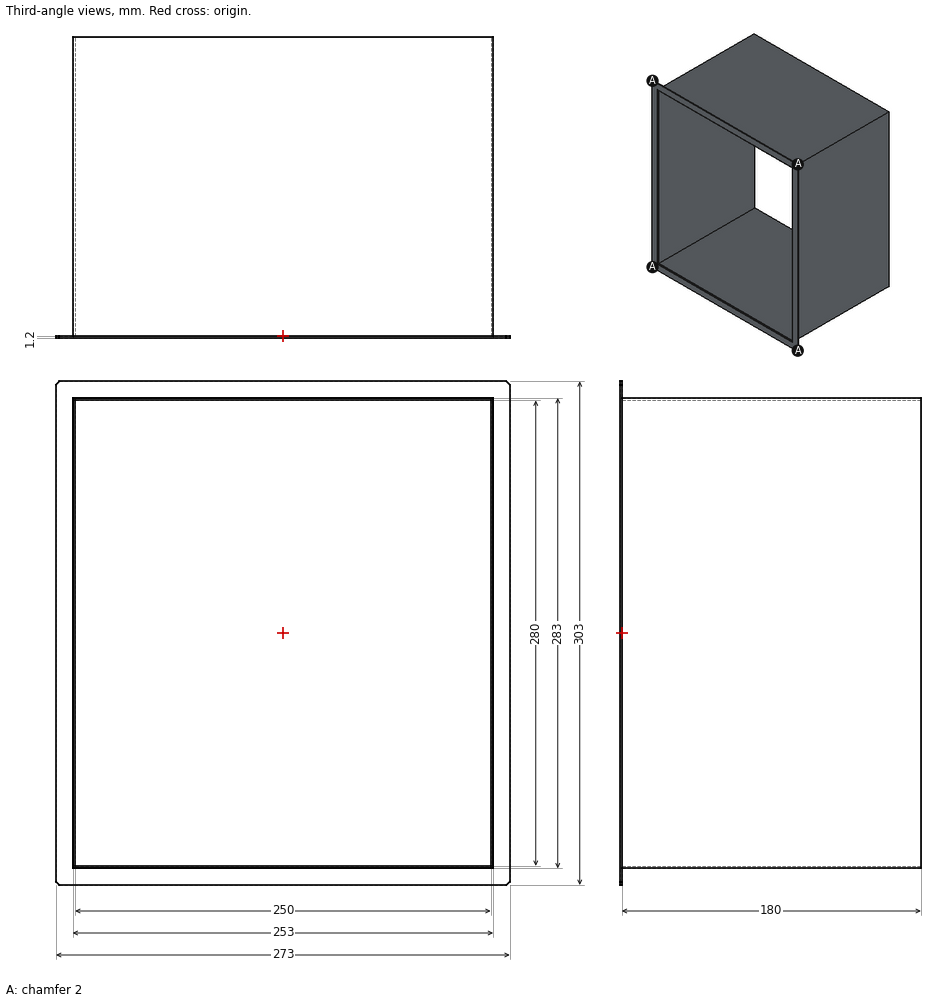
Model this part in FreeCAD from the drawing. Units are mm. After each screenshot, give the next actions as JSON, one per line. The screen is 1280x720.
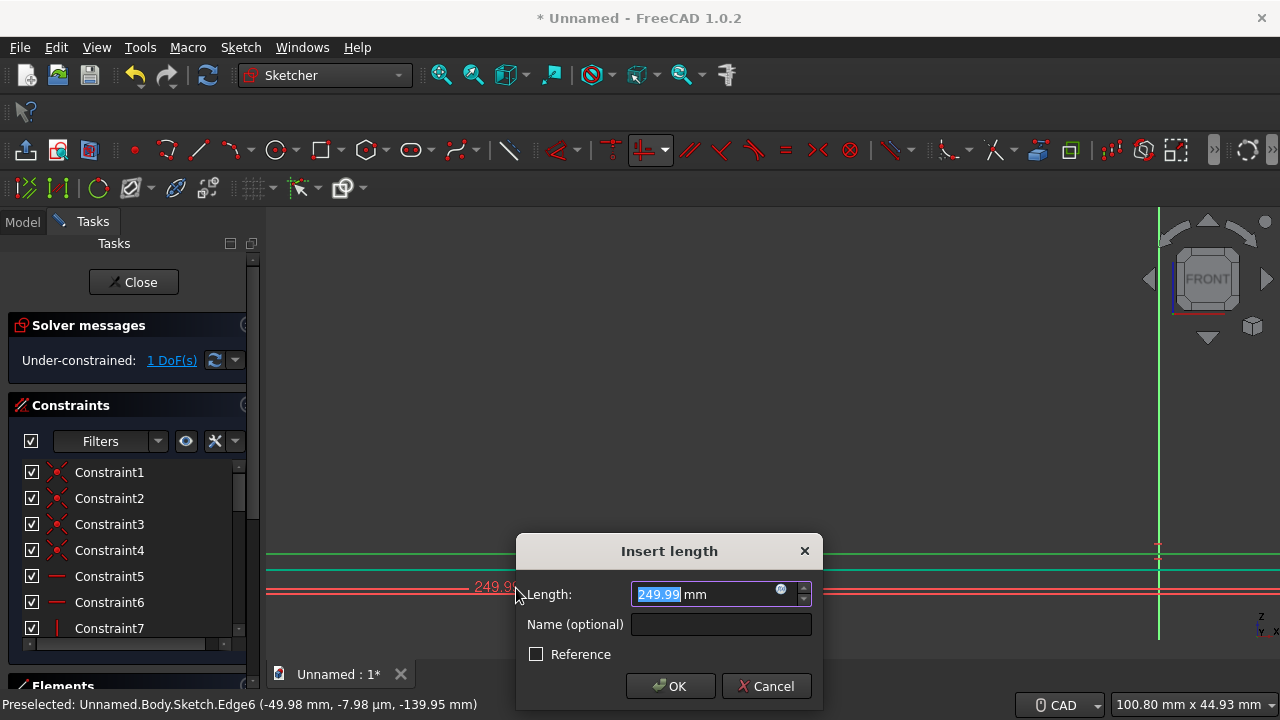
{"action": "type", "text": "250"}
{"action": "key", "text": "Return"}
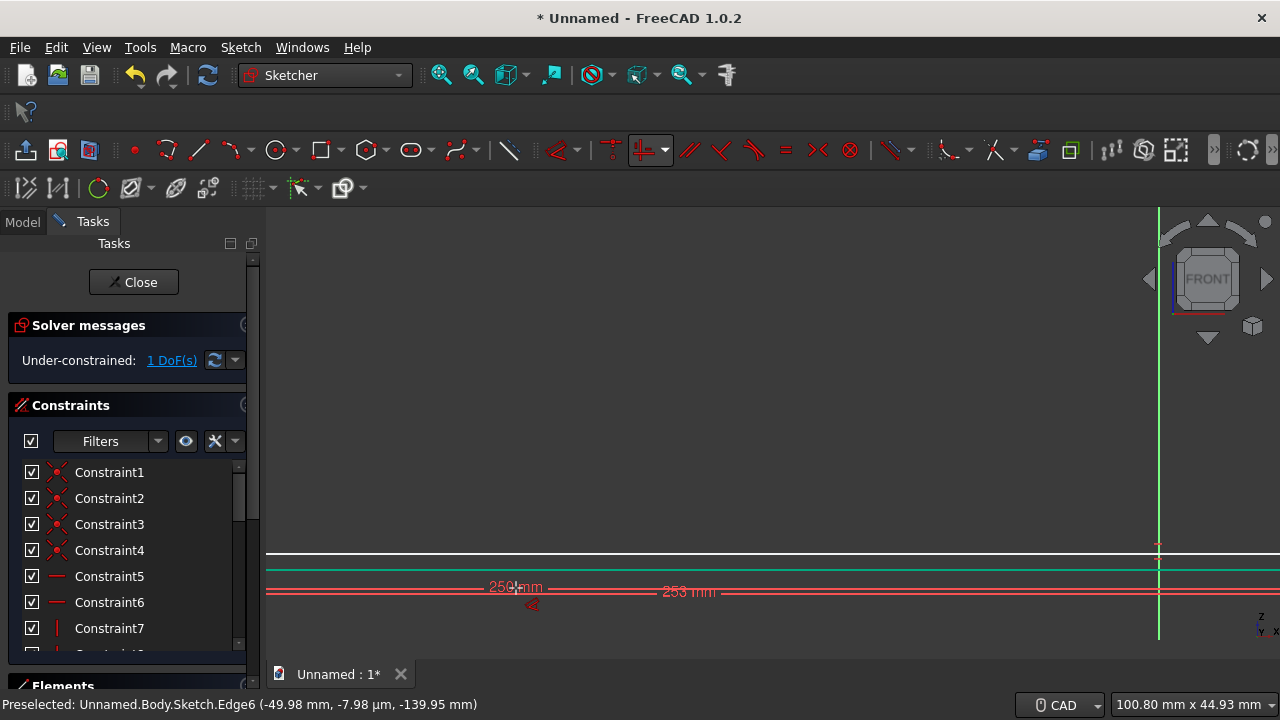
{"action": "scroll", "coordinate": [659, 561], "scroll_direction": "down", "scroll_amount": 12}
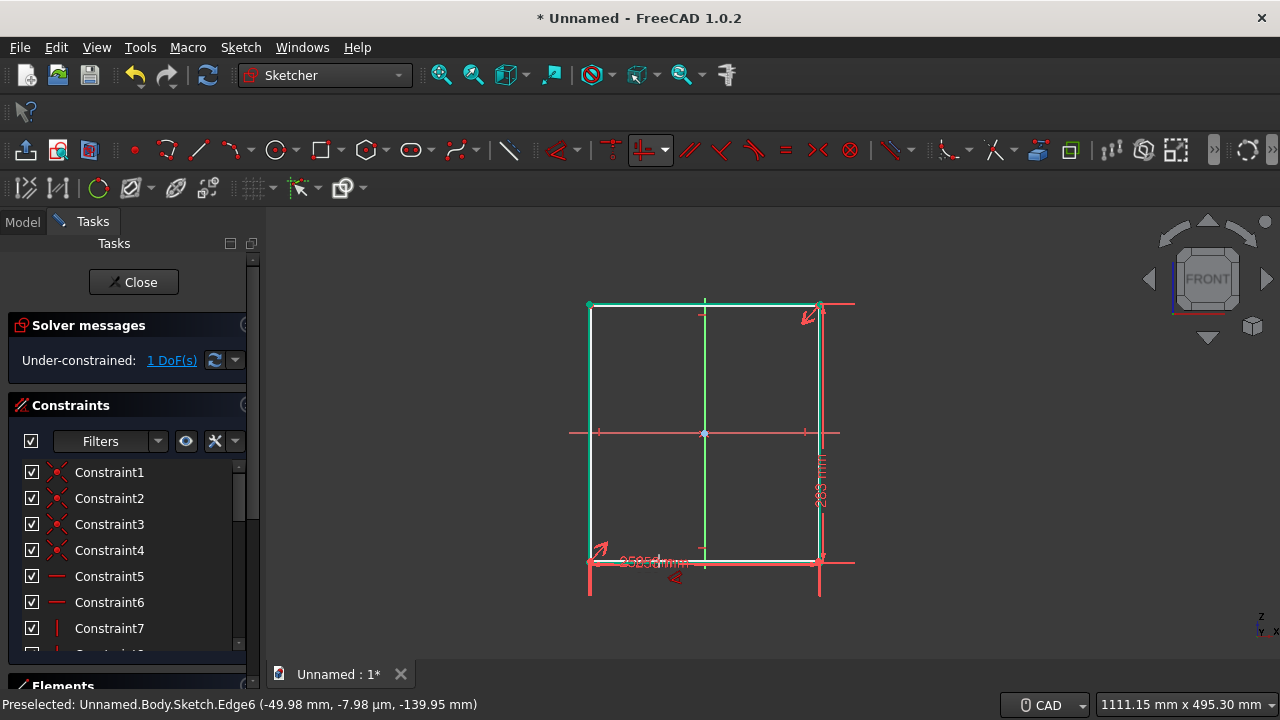
{"action": "scroll", "coordinate": [819, 484], "scroll_direction": "up", "scroll_amount": 12}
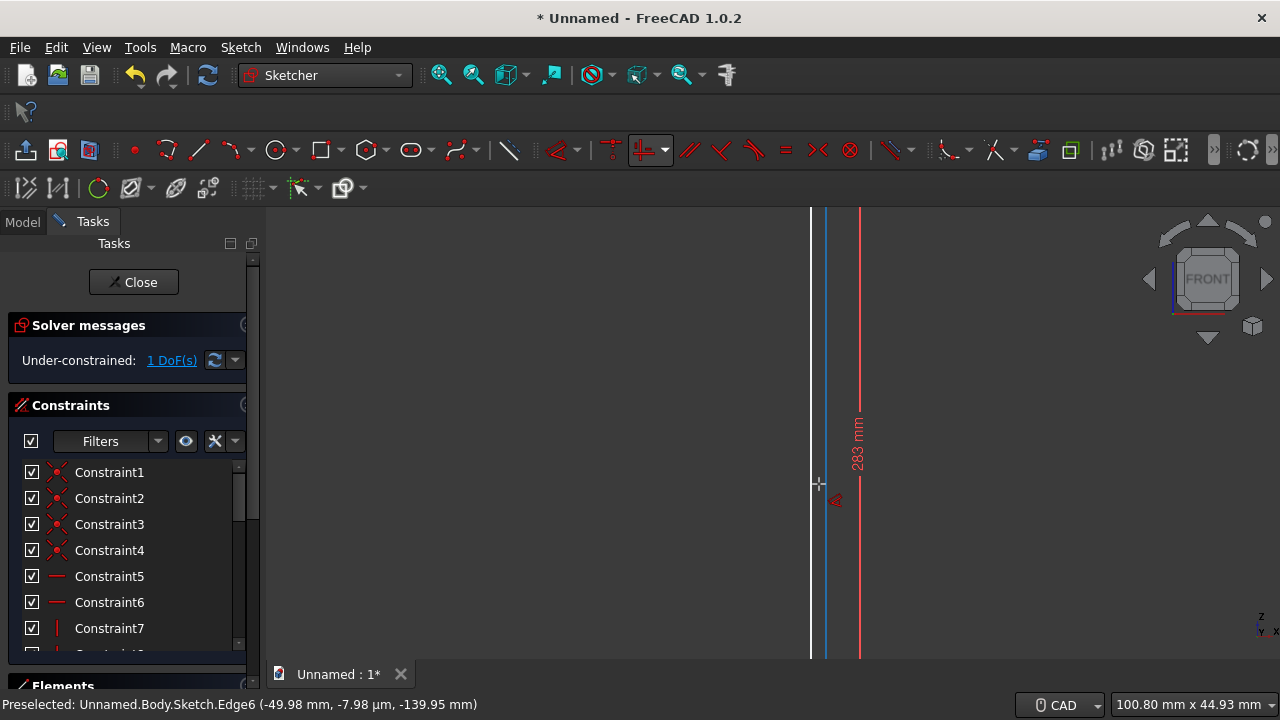
{"action": "left_click", "coordinate": [811, 483]}
{"action": "left_click", "coordinate": [845, 342]}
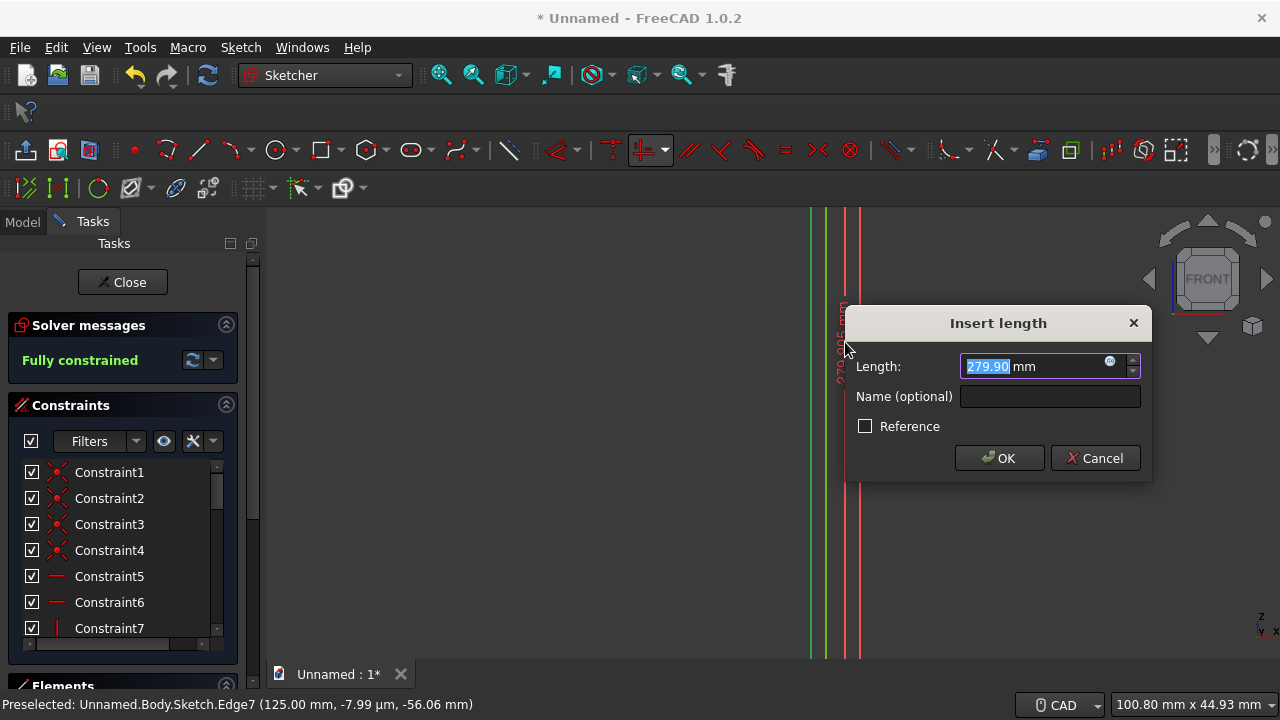
{"action": "type", "text": "280"}
{"action": "key", "text": "Return"}
{"action": "key", "text": "Escape"}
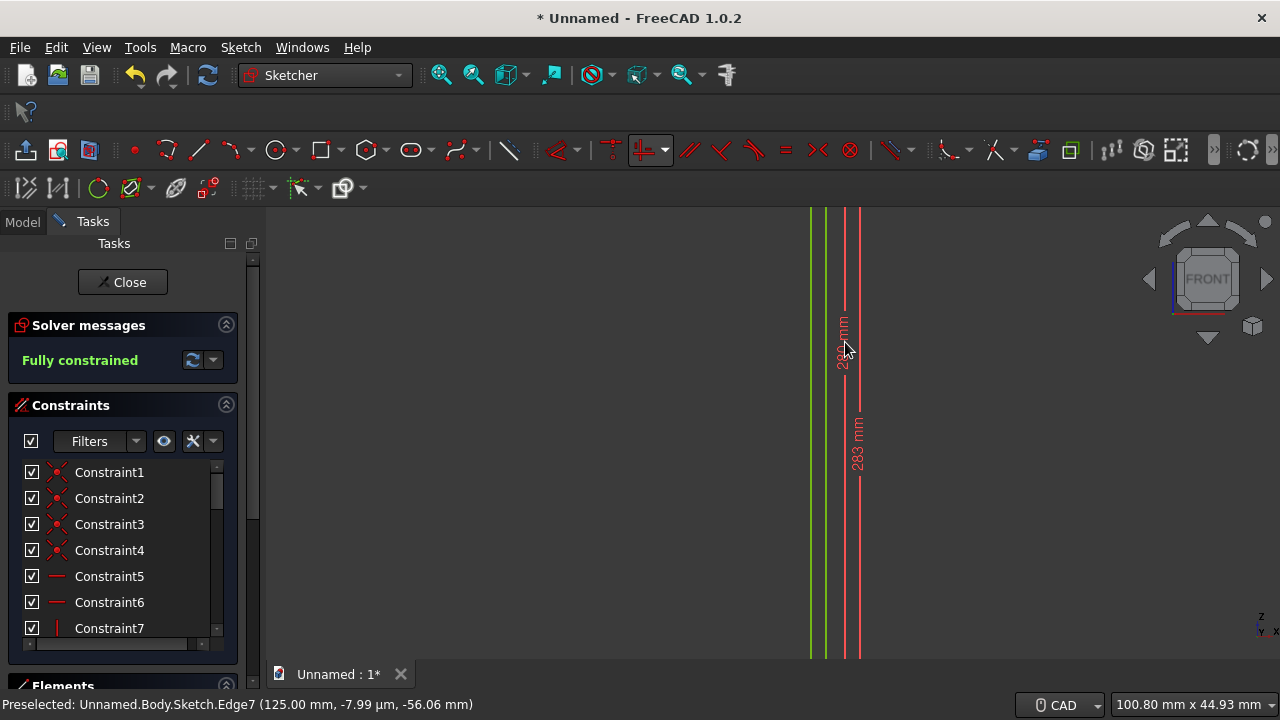
{"action": "left_click", "coordinate": [123, 282]}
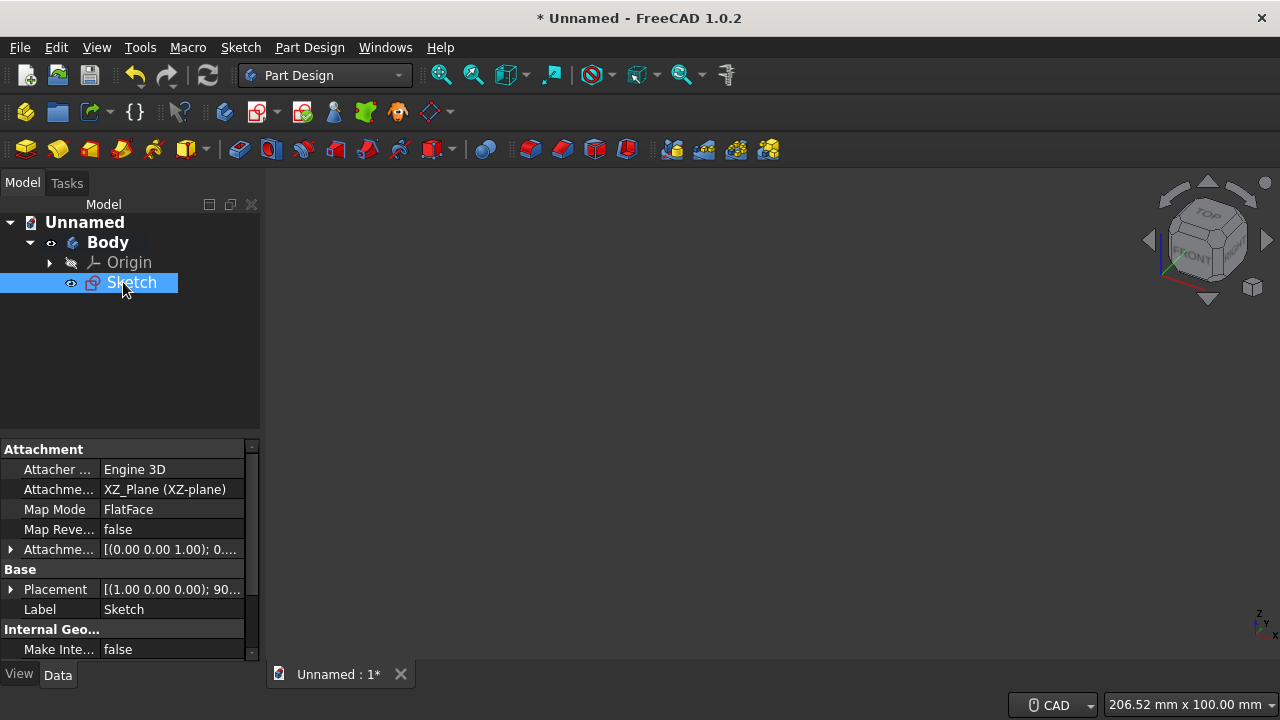
{"action": "left_click", "coordinate": [26, 150]}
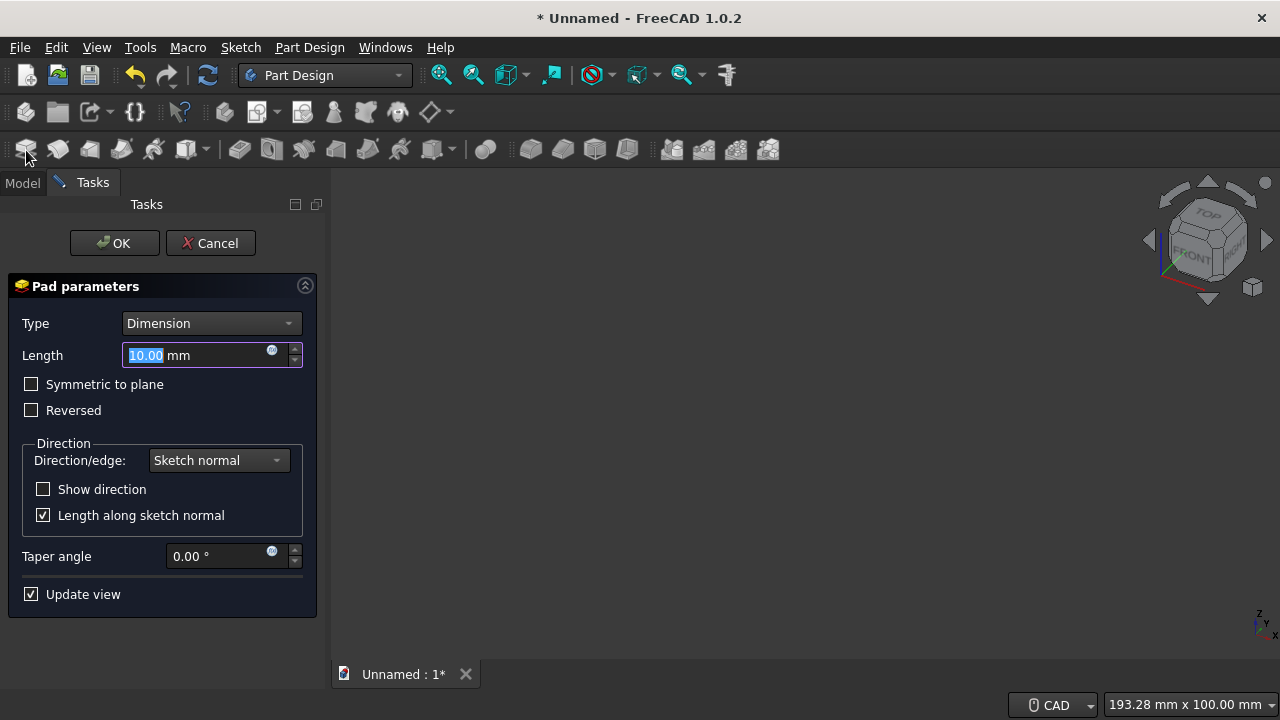
{"action": "type", "text": "180"}
{"action": "key", "text": "Tab"}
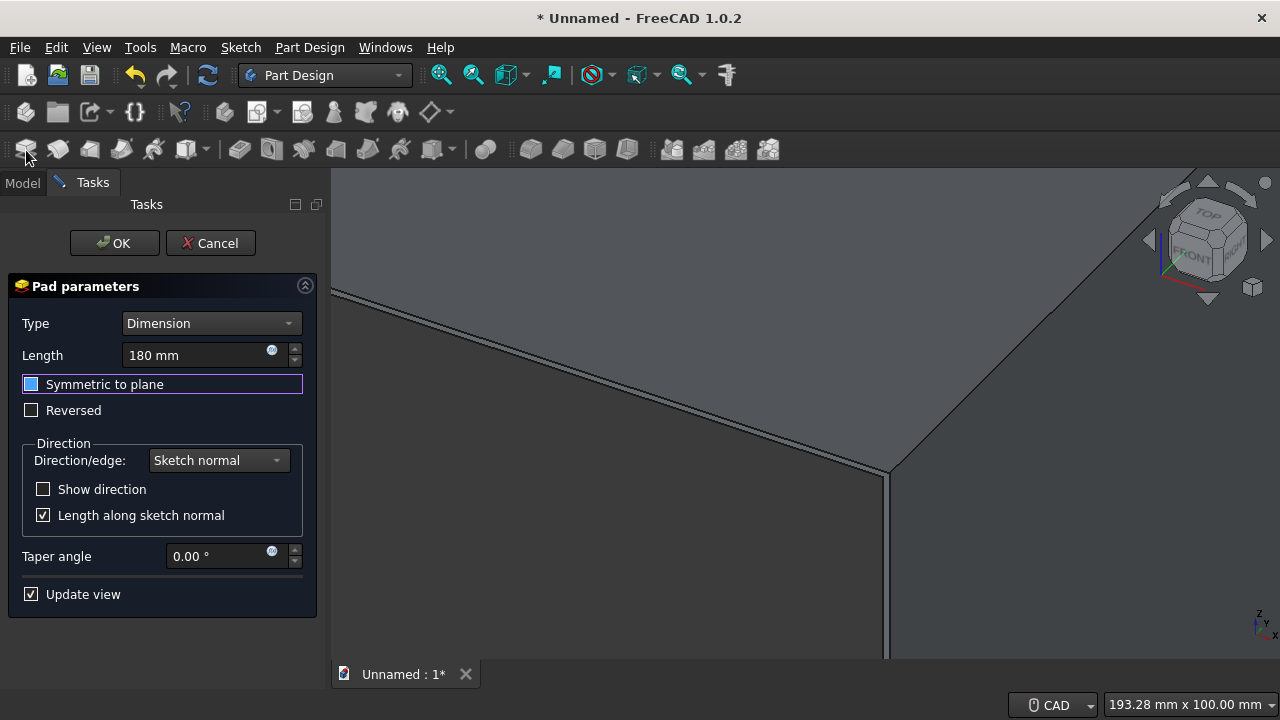
{"action": "left_click", "coordinate": [30, 410]}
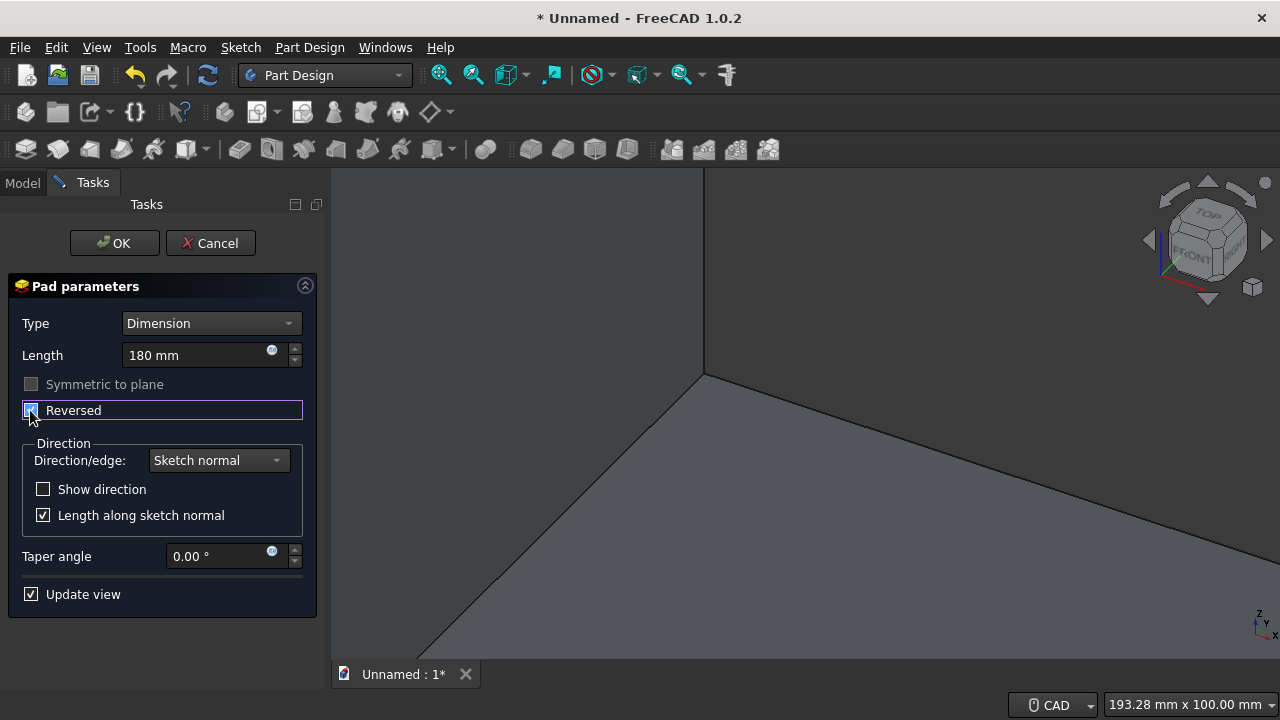
{"action": "left_click", "coordinate": [115, 243]}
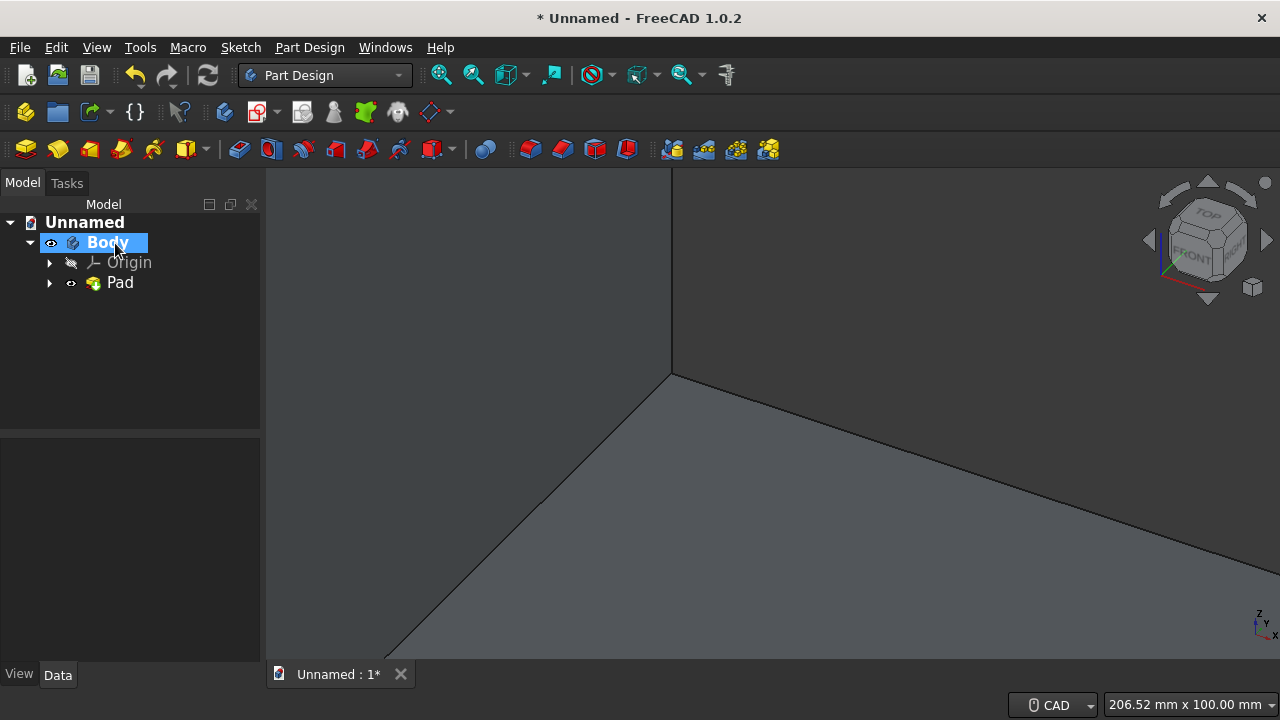
{"action": "key", "text": "v f"}